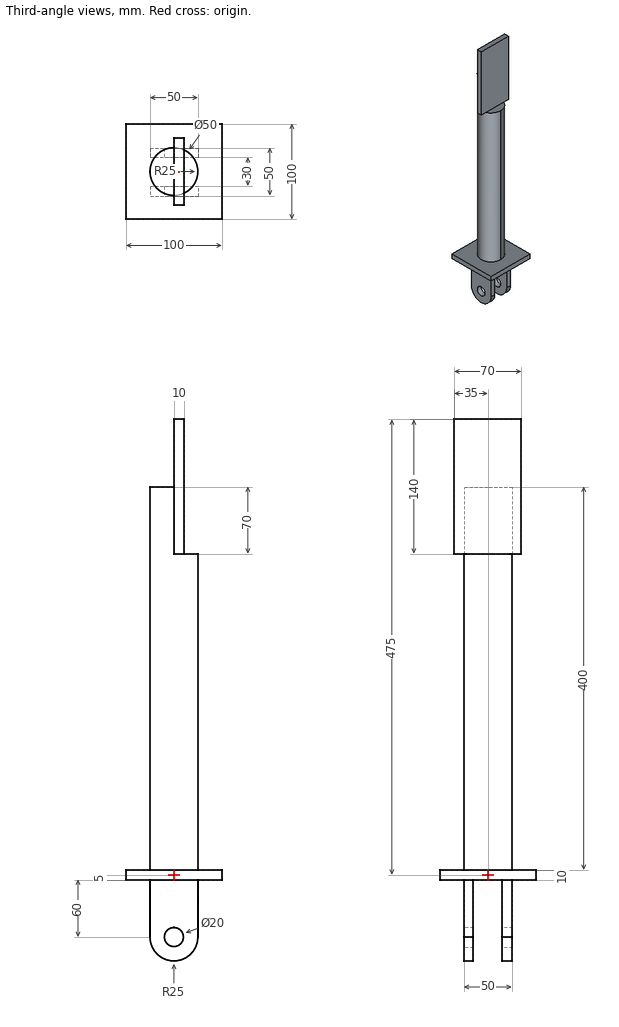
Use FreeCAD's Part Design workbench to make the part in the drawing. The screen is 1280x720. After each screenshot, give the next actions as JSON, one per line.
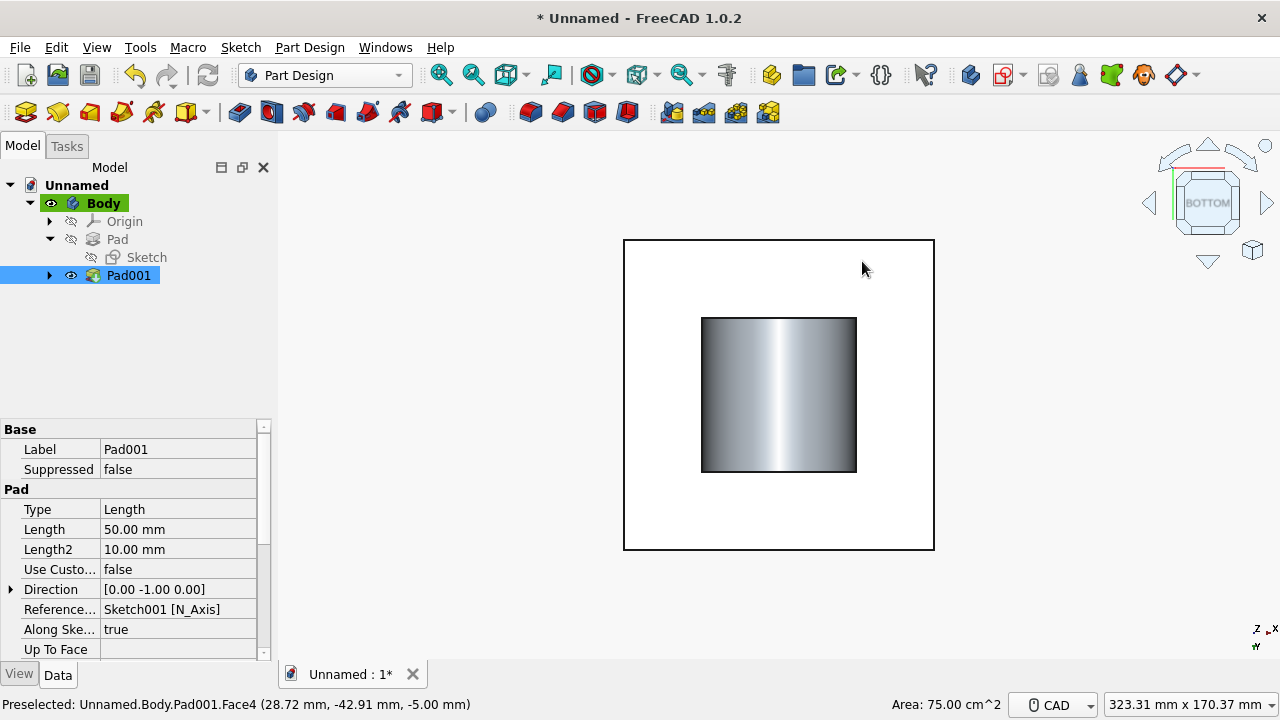
{"action": "left_click", "coordinate": [1004, 76]}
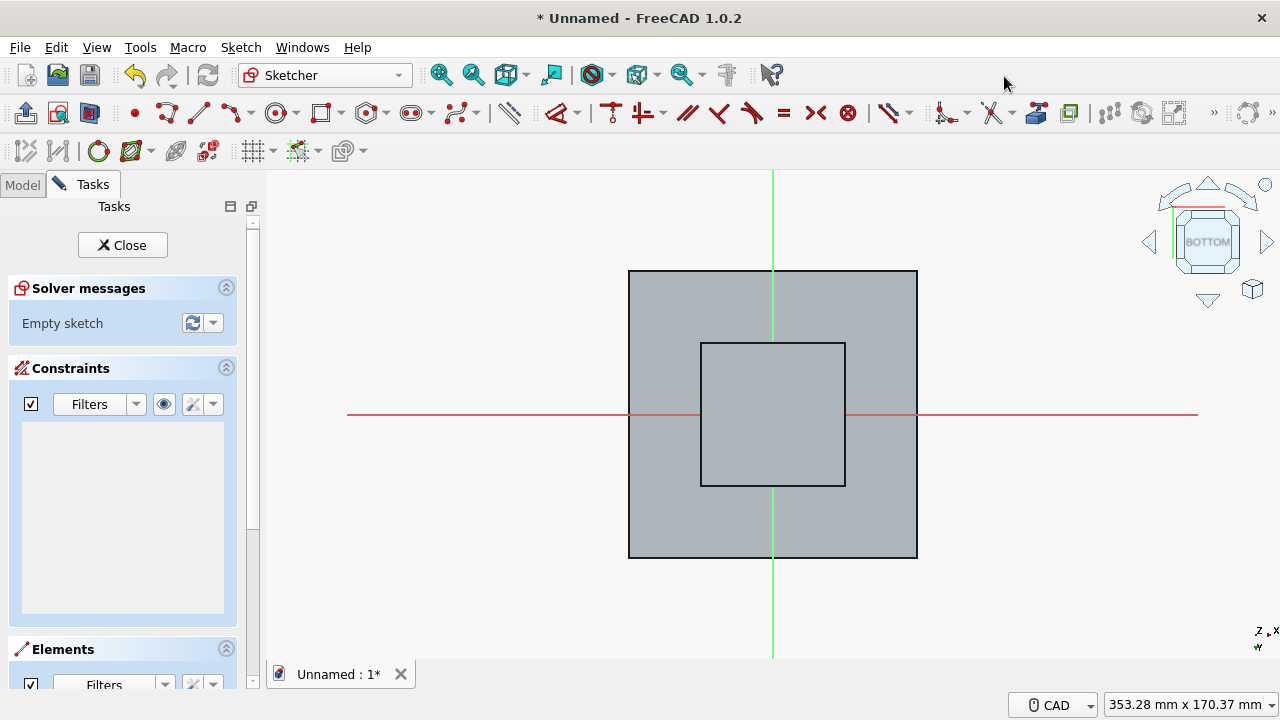
{"action": "scroll", "coordinate": [803, 415], "scroll_direction": "up", "scroll_amount": 6}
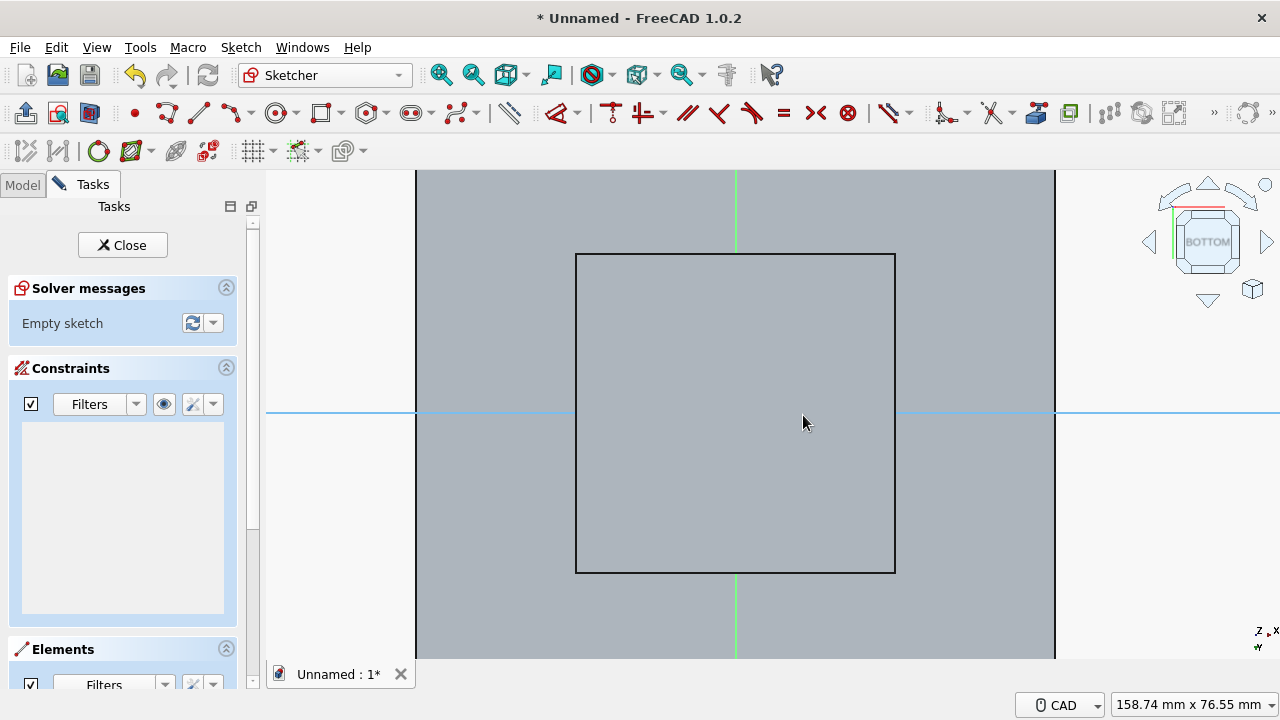
{"action": "key", "text": "g v"}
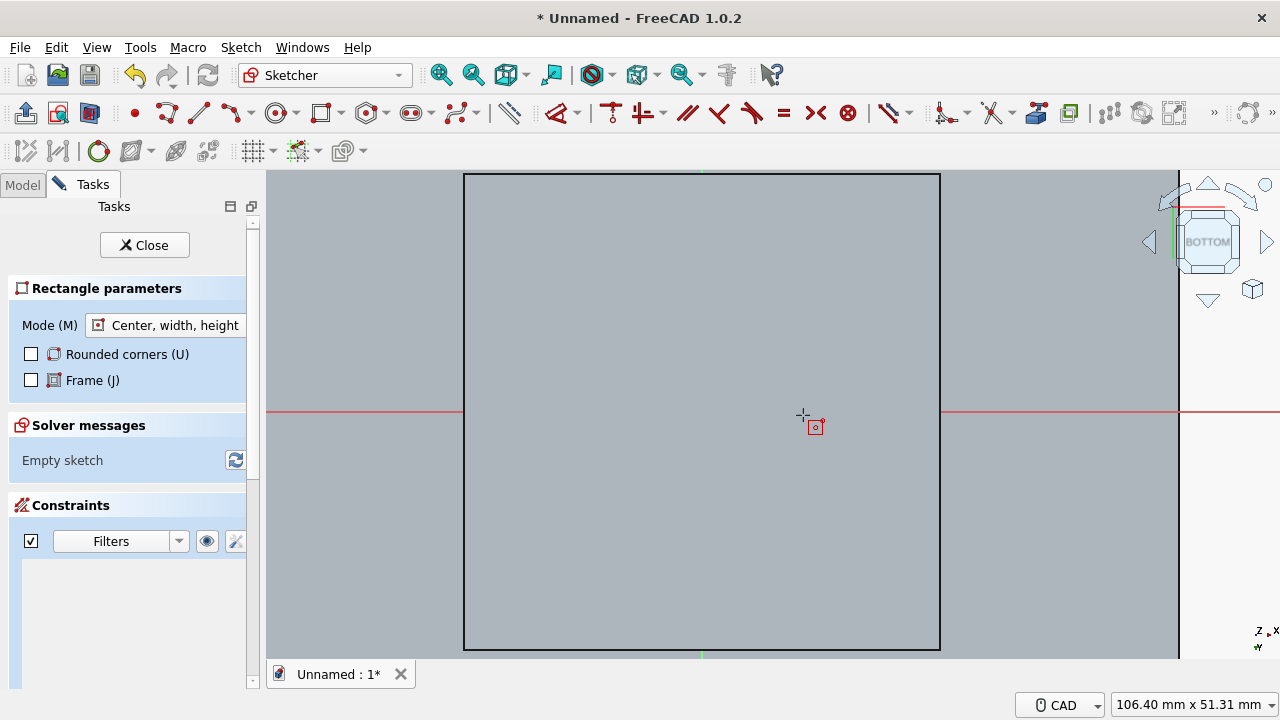
{"action": "left_click", "coordinate": [702, 412]}
{"action": "left_click", "coordinate": [940, 269]}
{"action": "key", "text": "Escape"}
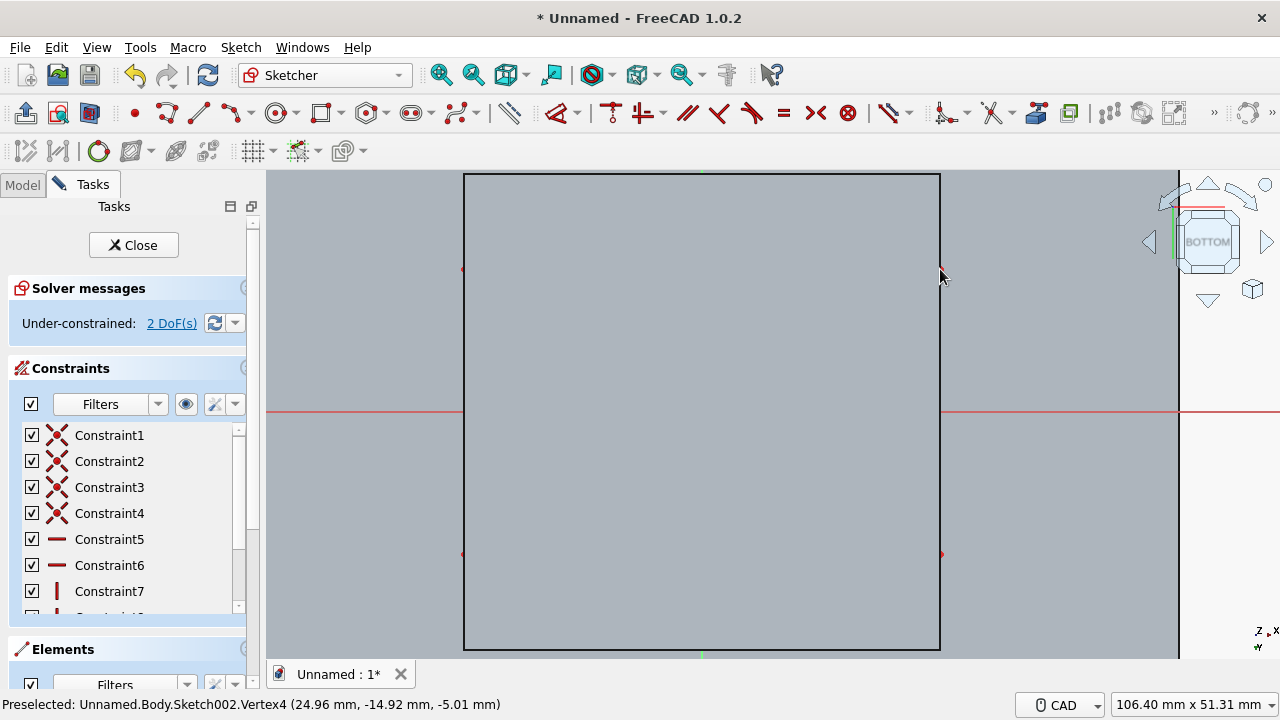
{"action": "key", "text": "d"}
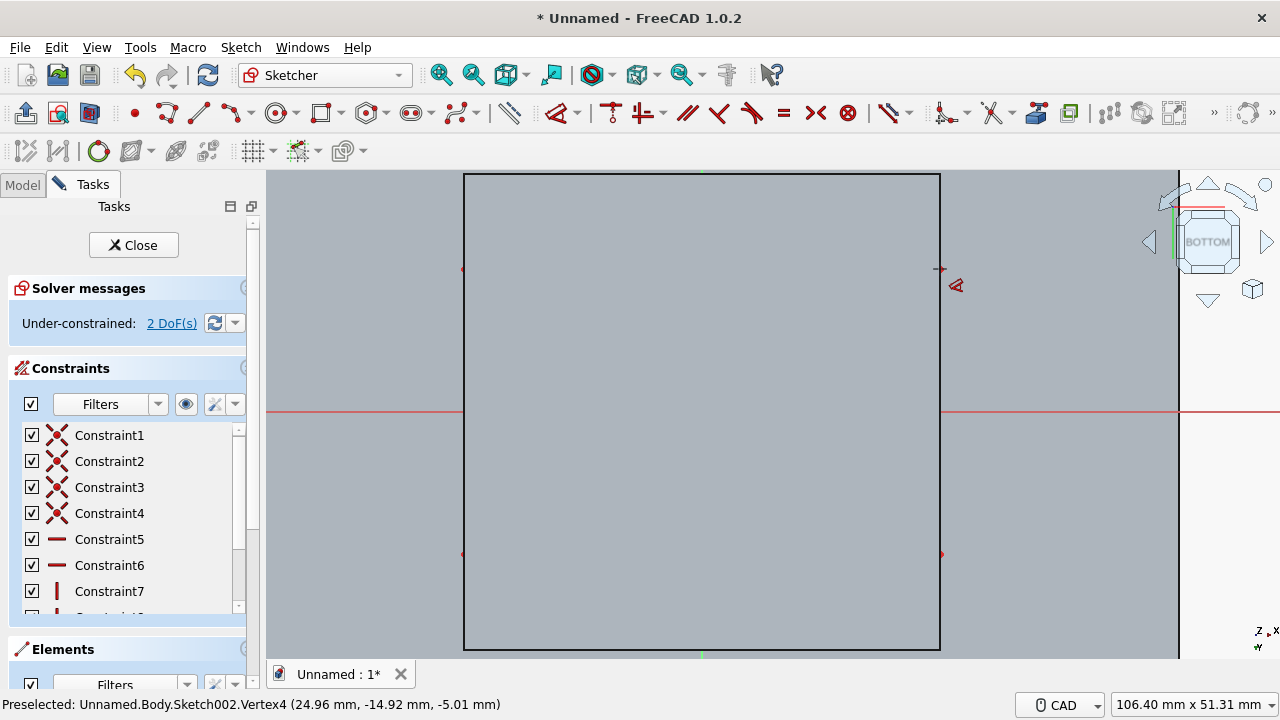
{"action": "left_click", "coordinate": [607, 554]}
{"action": "left_click", "coordinate": [593, 588]}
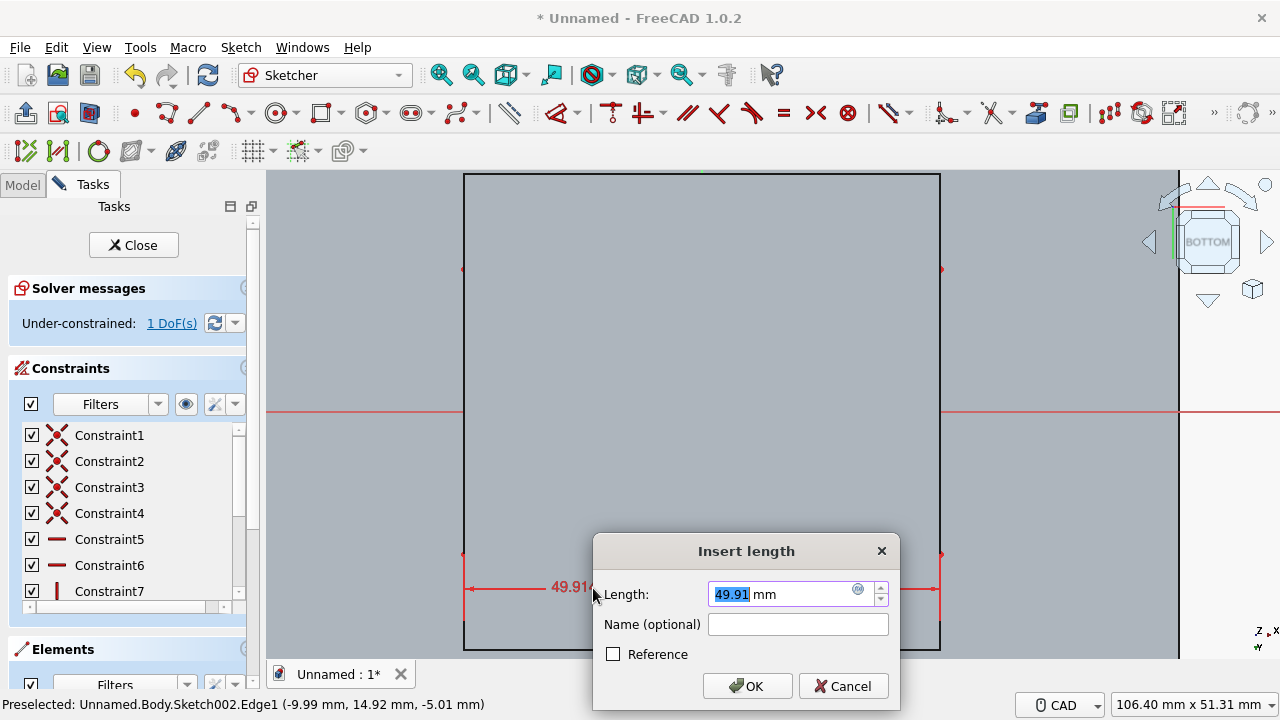
{"action": "type", "text": "50"}
{"action": "key", "text": "Return"}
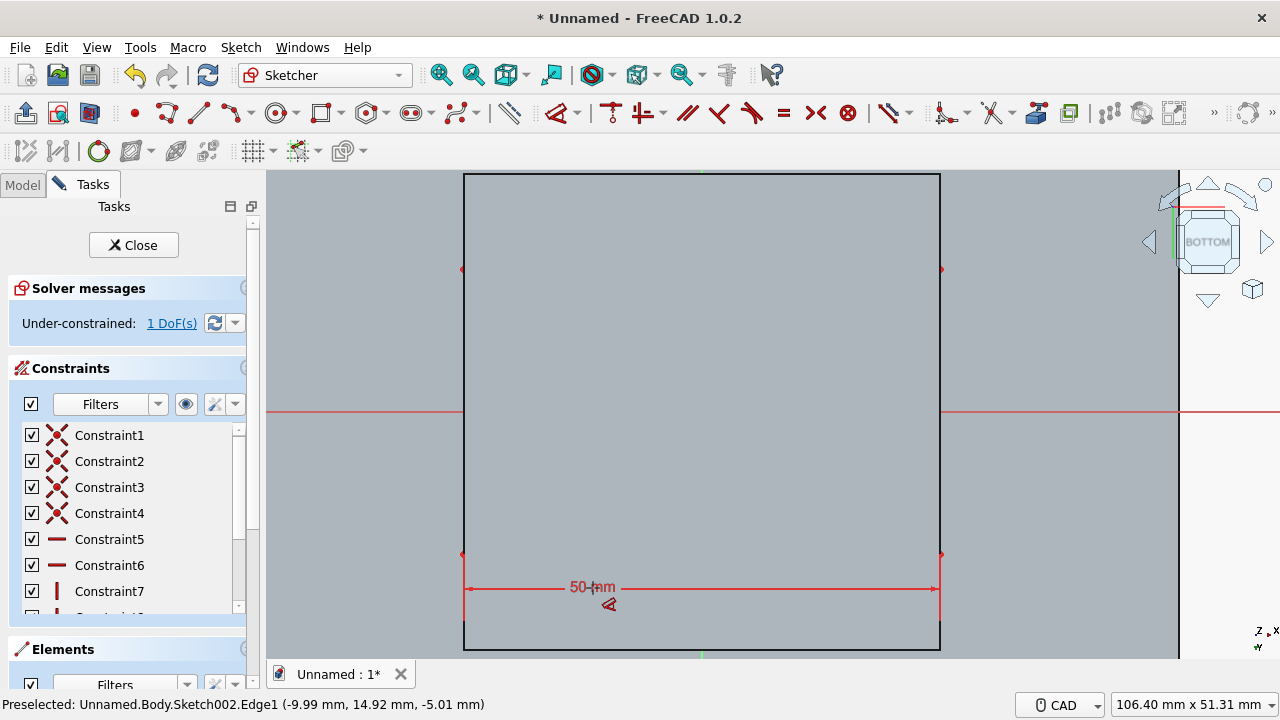
{"action": "left_click", "coordinate": [940, 469]}
{"action": "left_click", "coordinate": [974, 347]}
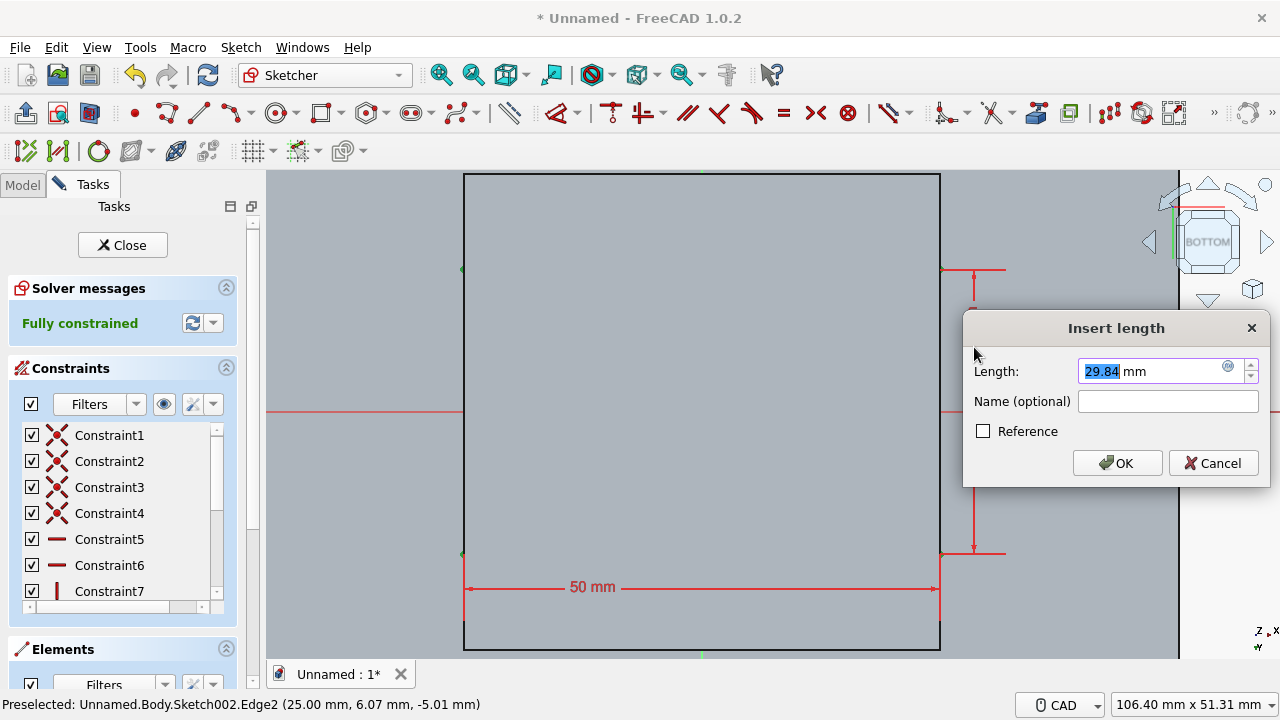
{"action": "type", "text": "30"}
{"action": "key", "text": "Return"}
{"action": "key", "text": "Escape"}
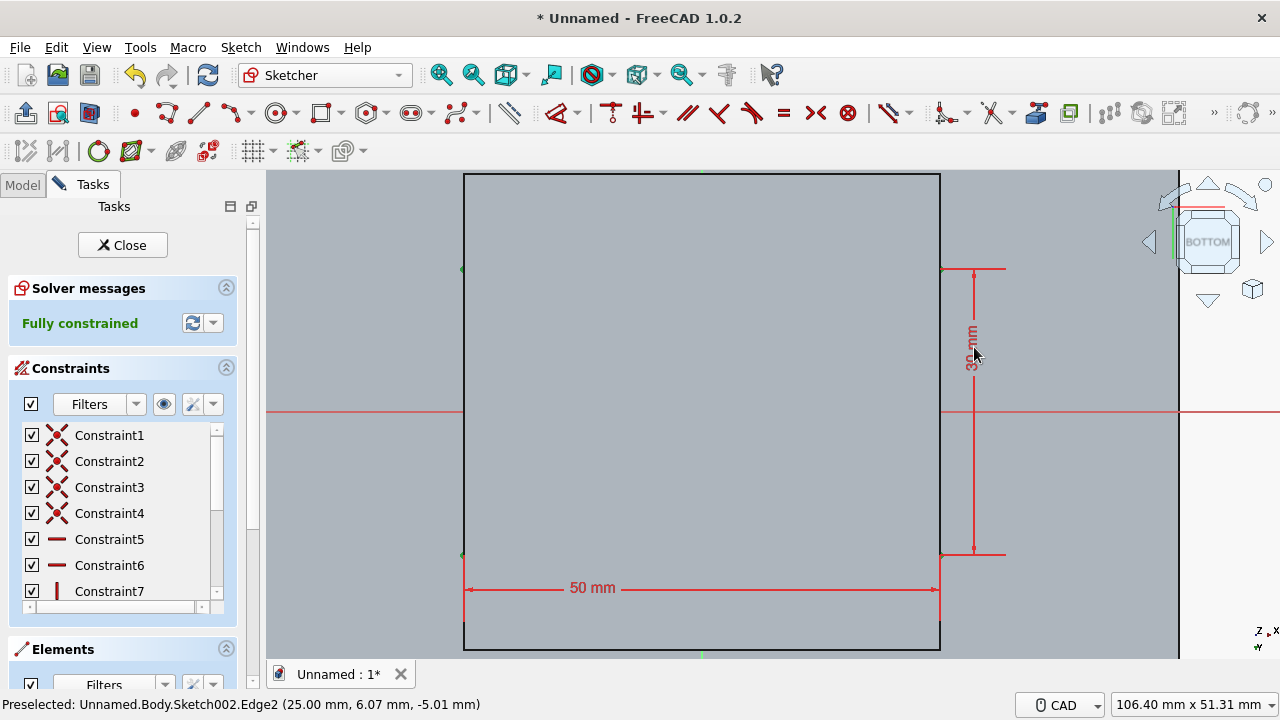
{"action": "left_click", "coordinate": [123, 245]}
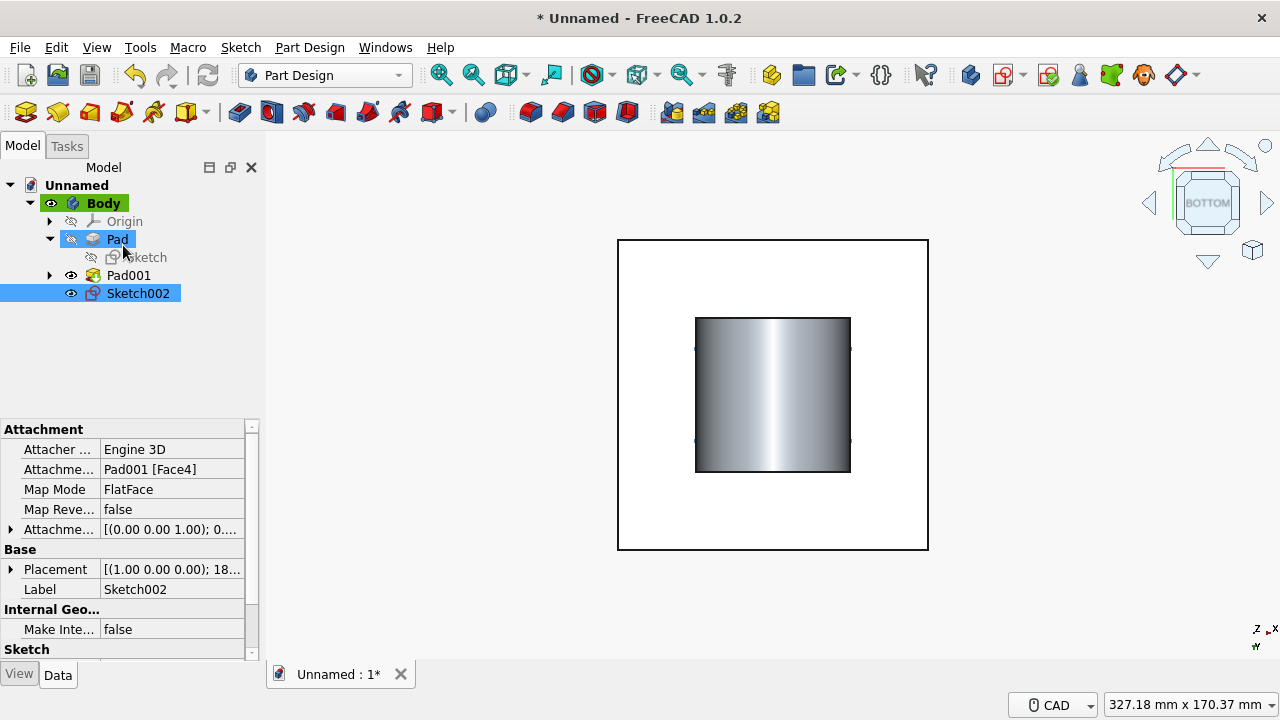
{"action": "left_click", "coordinate": [240, 112]}